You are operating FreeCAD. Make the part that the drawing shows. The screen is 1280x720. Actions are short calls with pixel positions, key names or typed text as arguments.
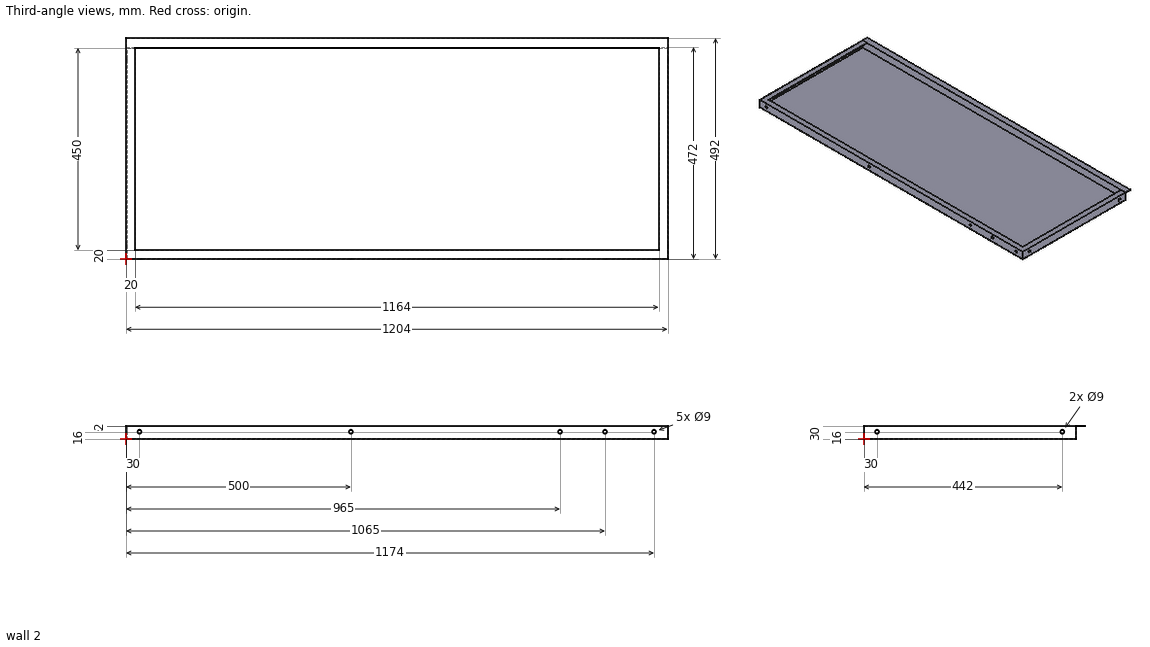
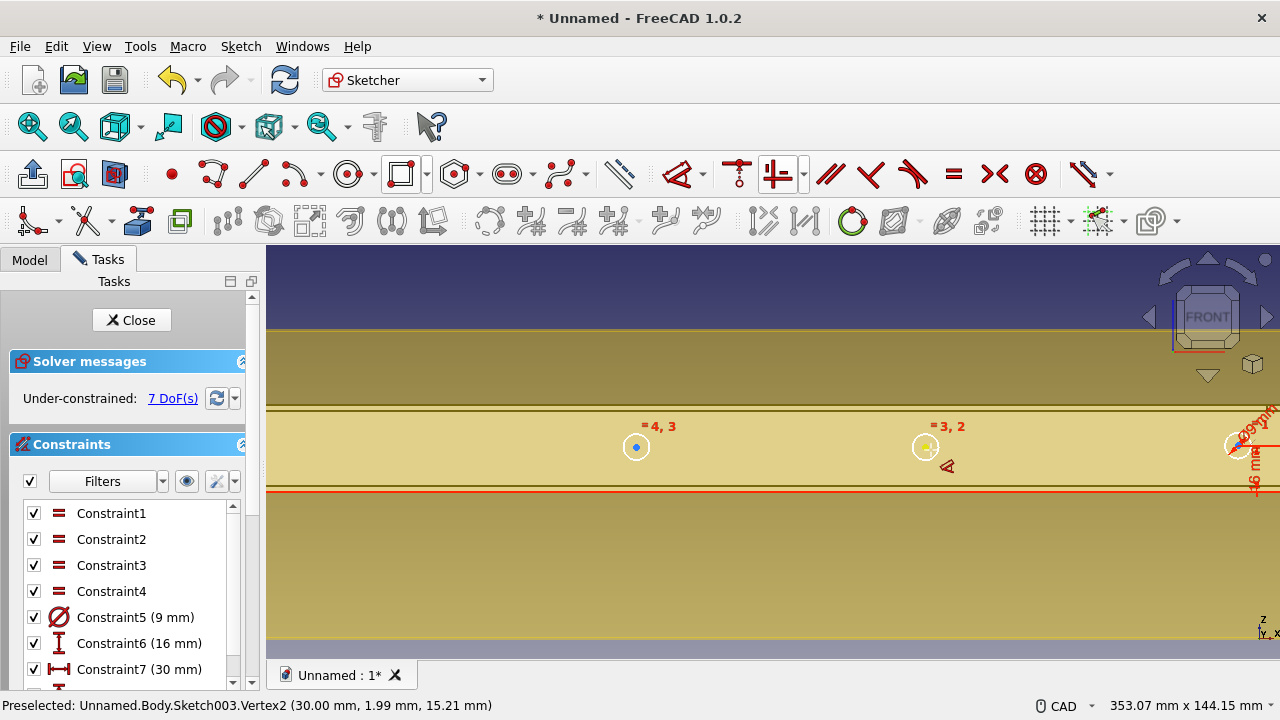
click(926, 447)
click(960, 469)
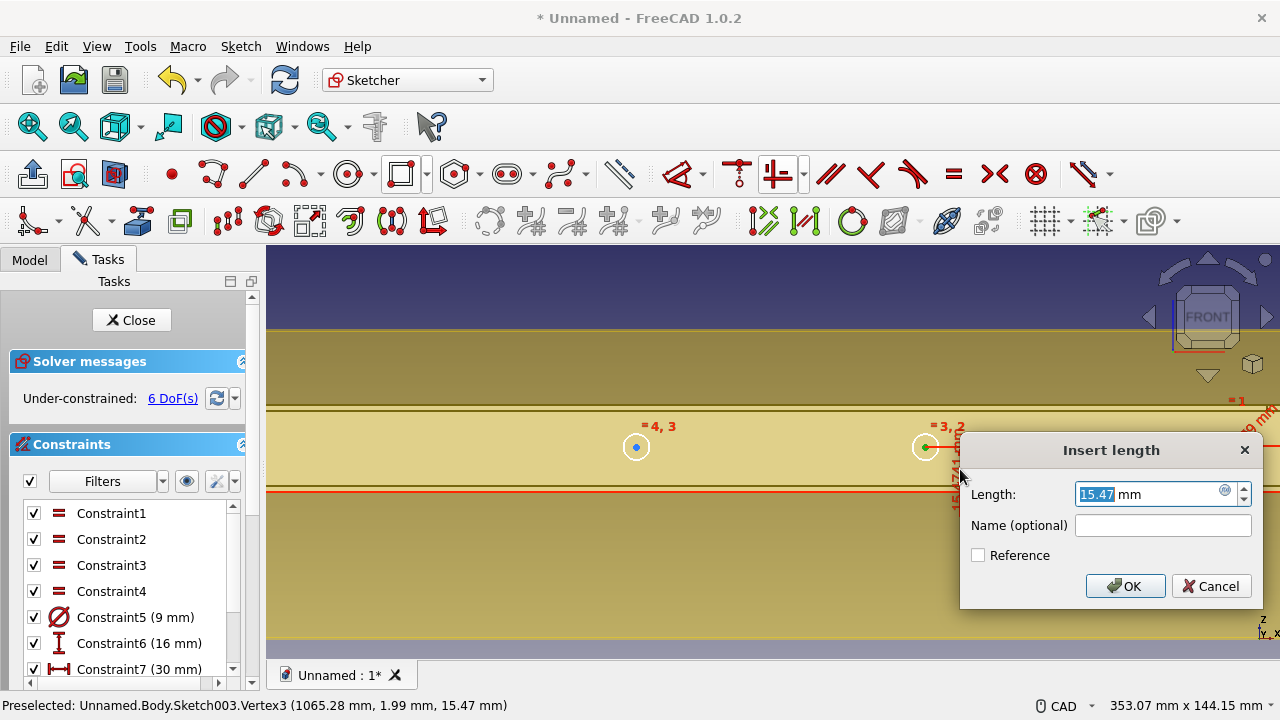
text(16)
key(Return)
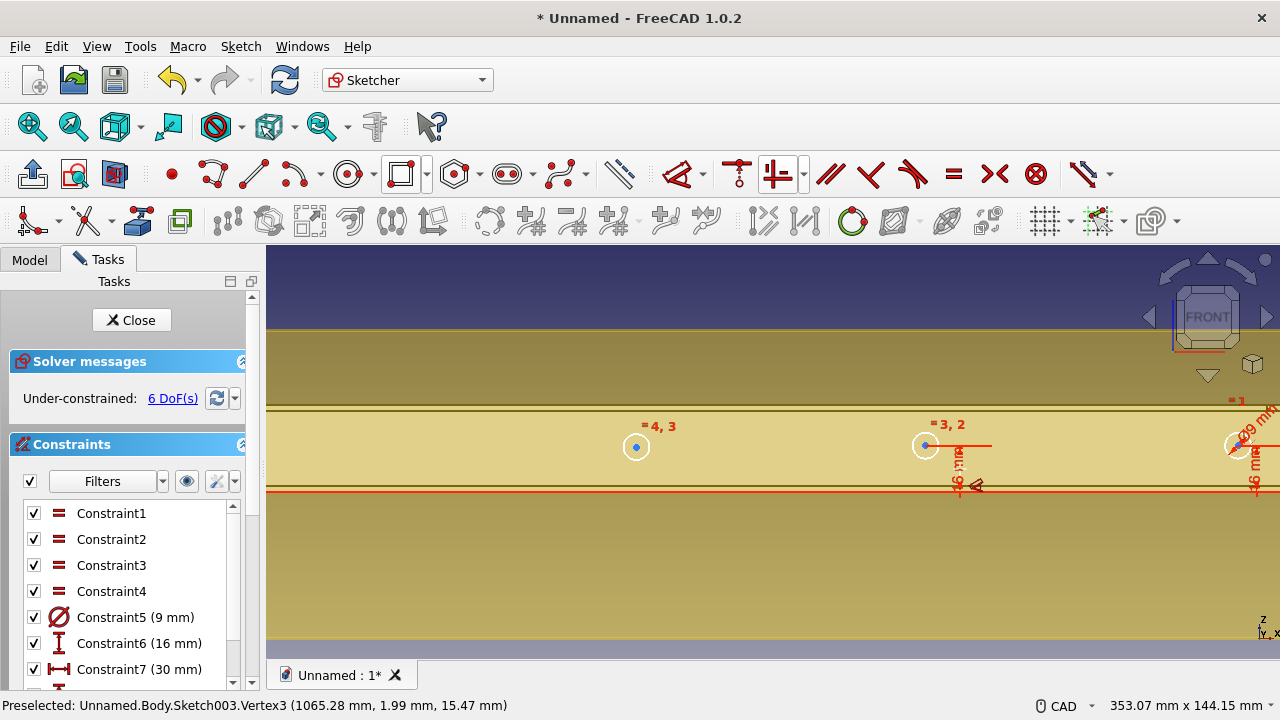
click(636, 447)
click(670, 469)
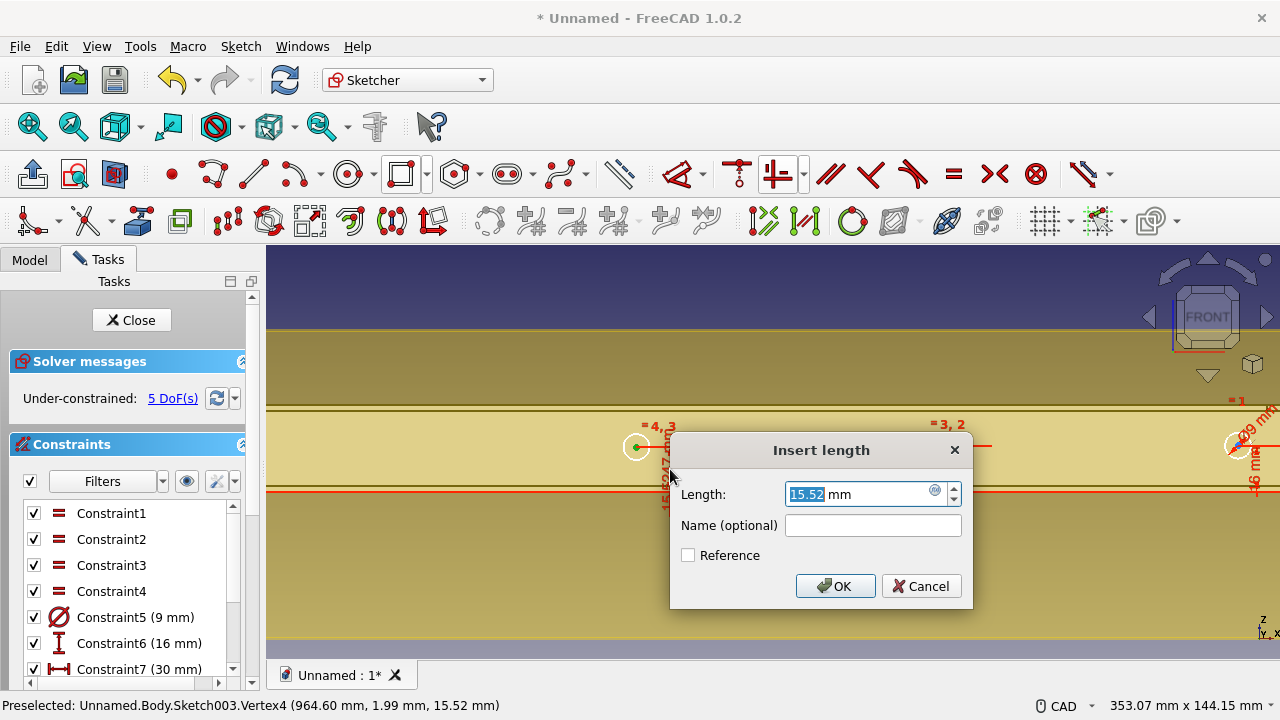
text(16)
key(Return)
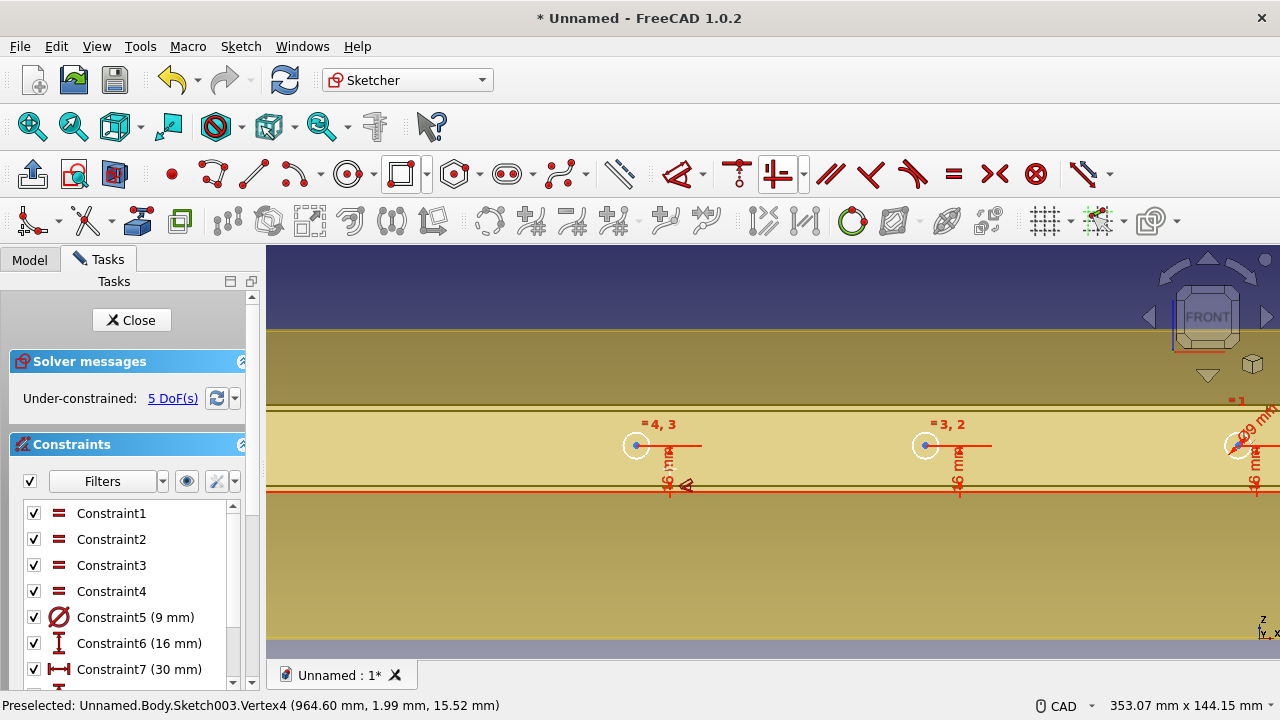
scroll(931, 450, down, 9)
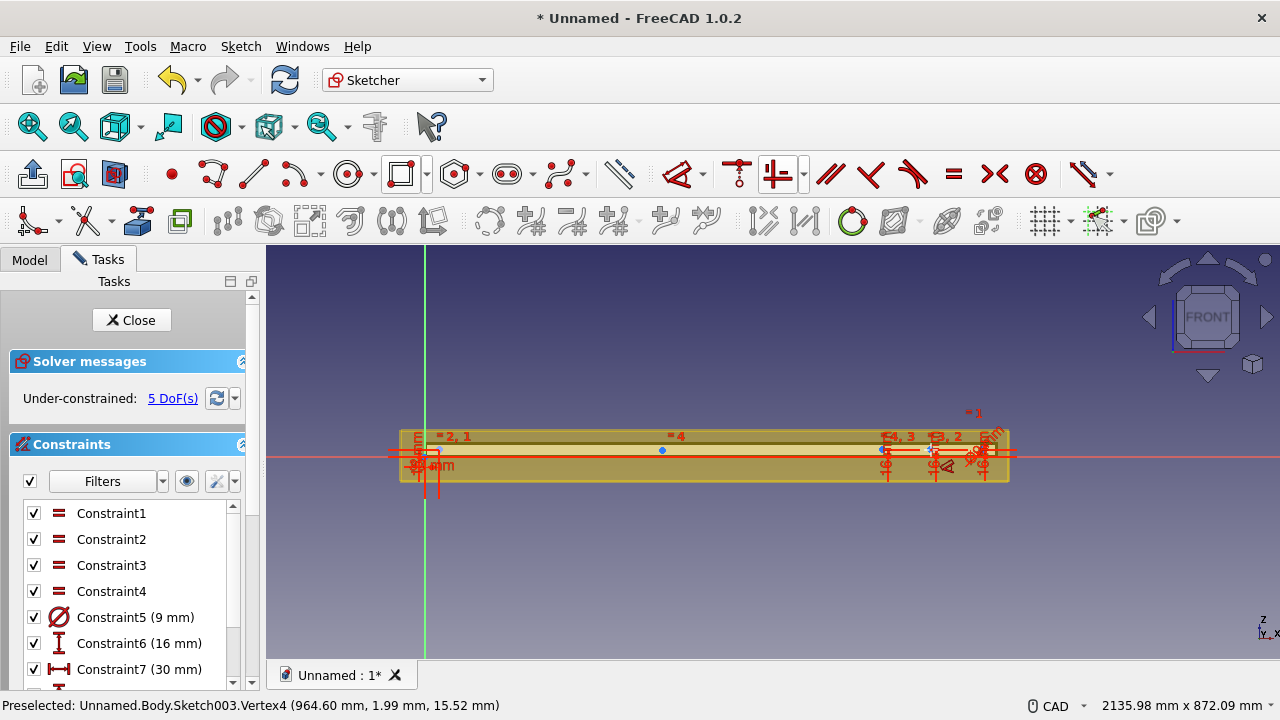
scroll(662, 450, up, 9)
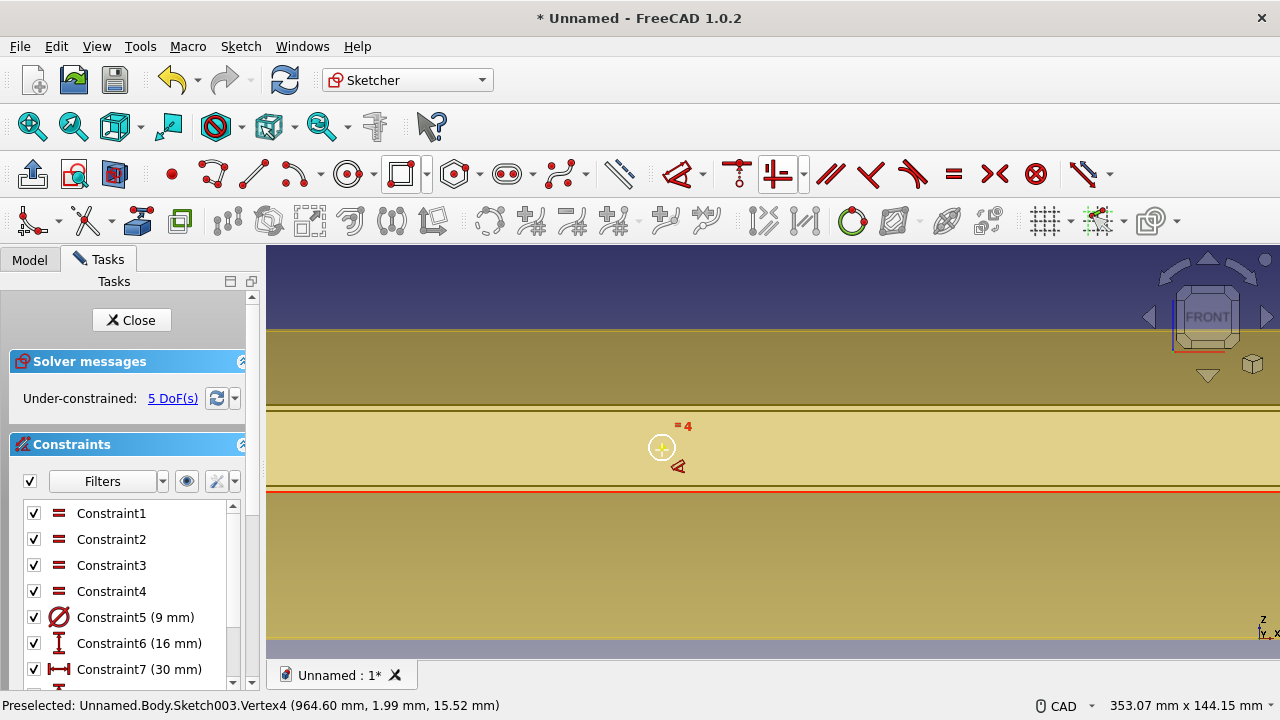
click(662, 448)
click(696, 470)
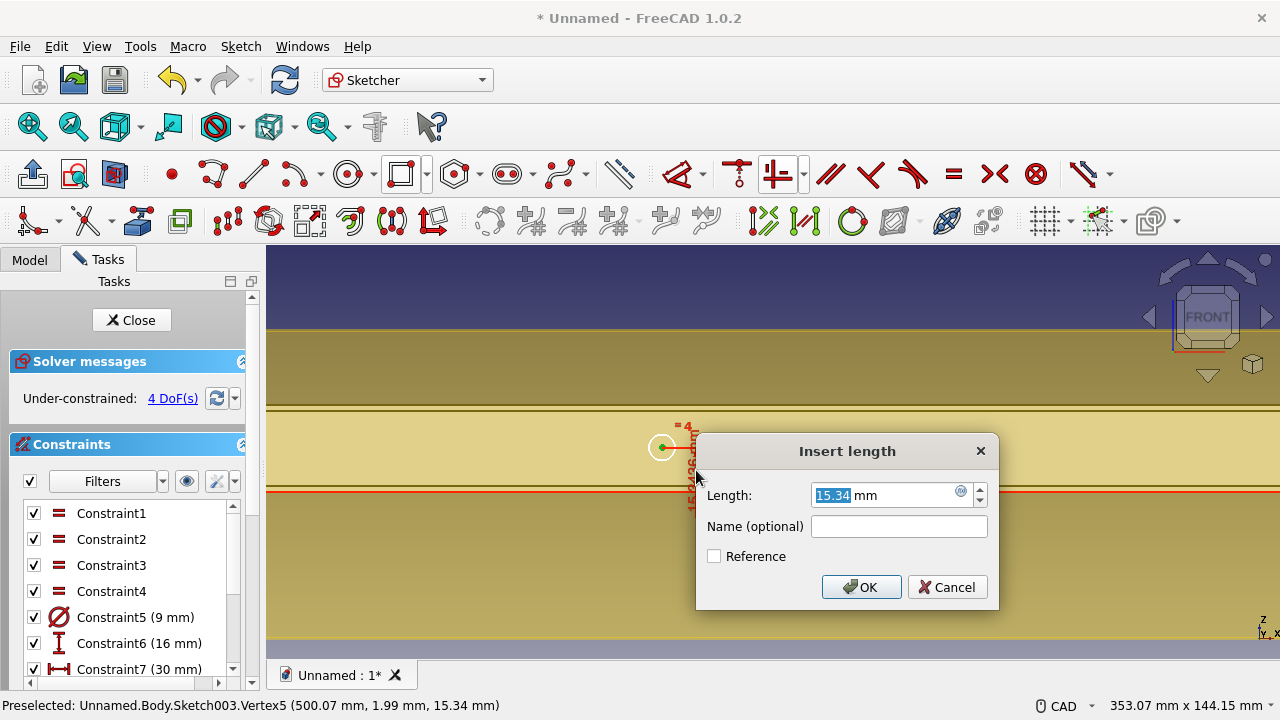
text(16)
key(Return)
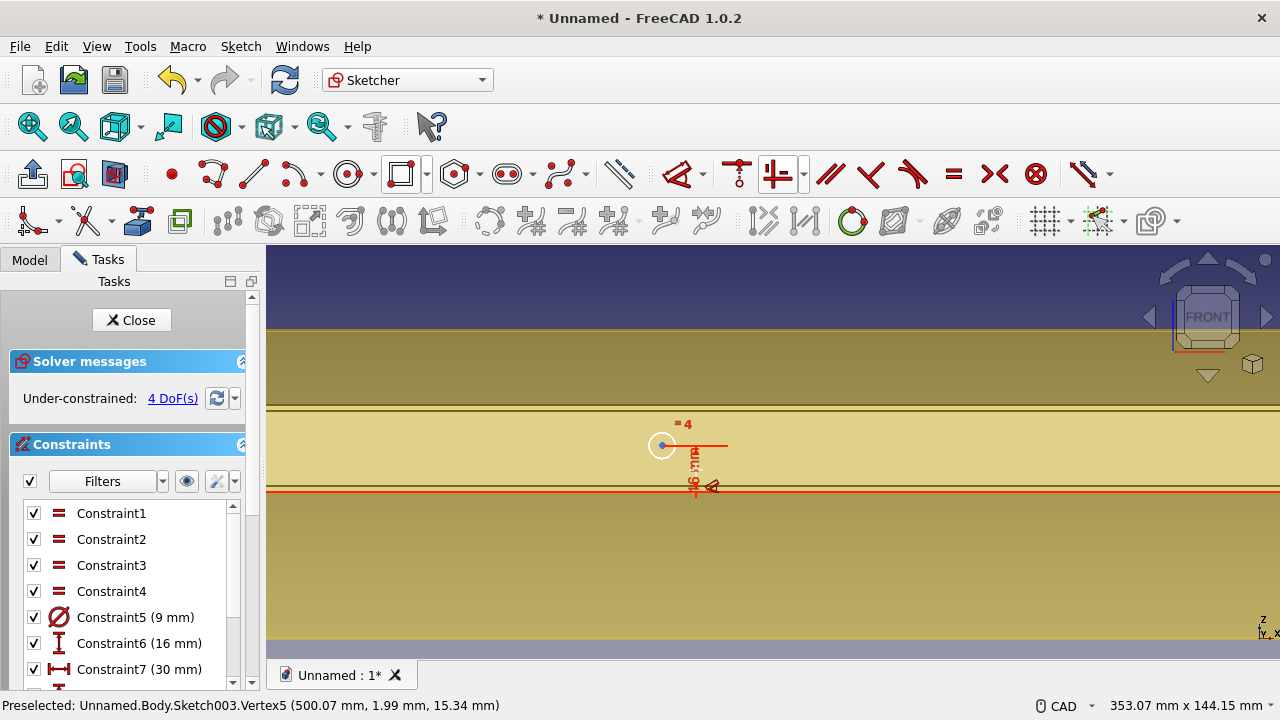
scroll(662, 450, down, 9)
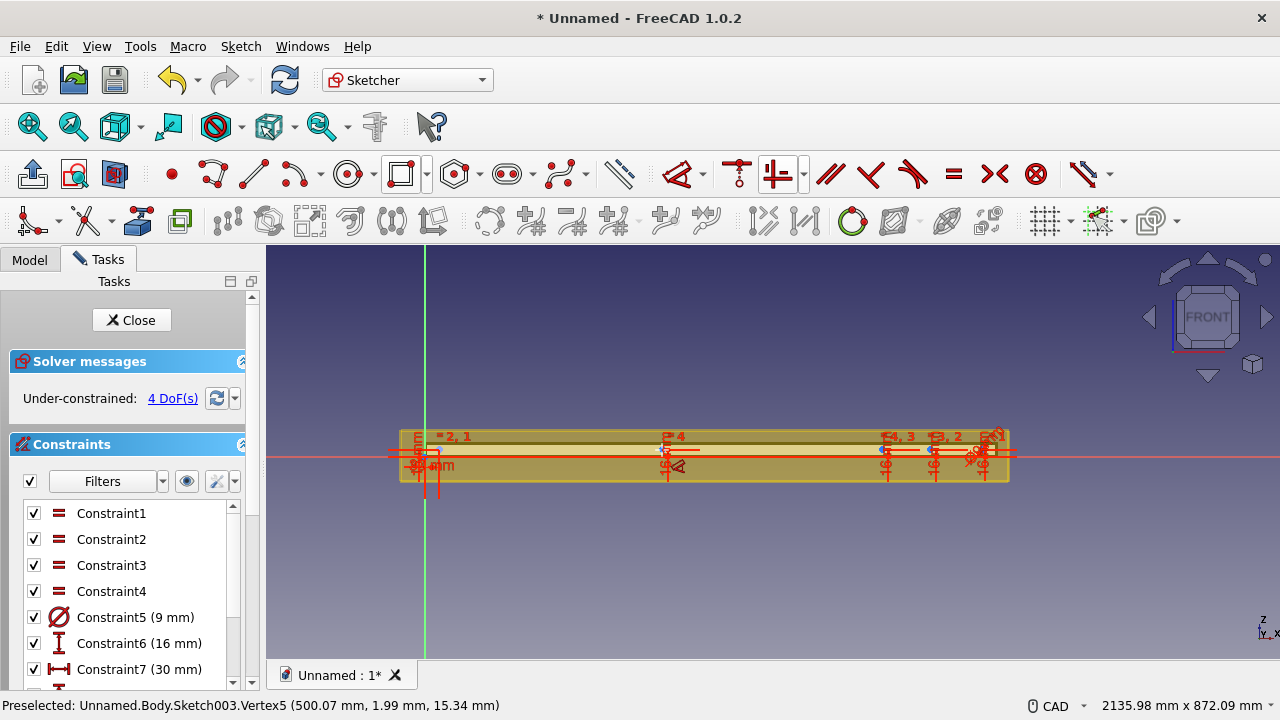
click(883, 450)
click(654, 491)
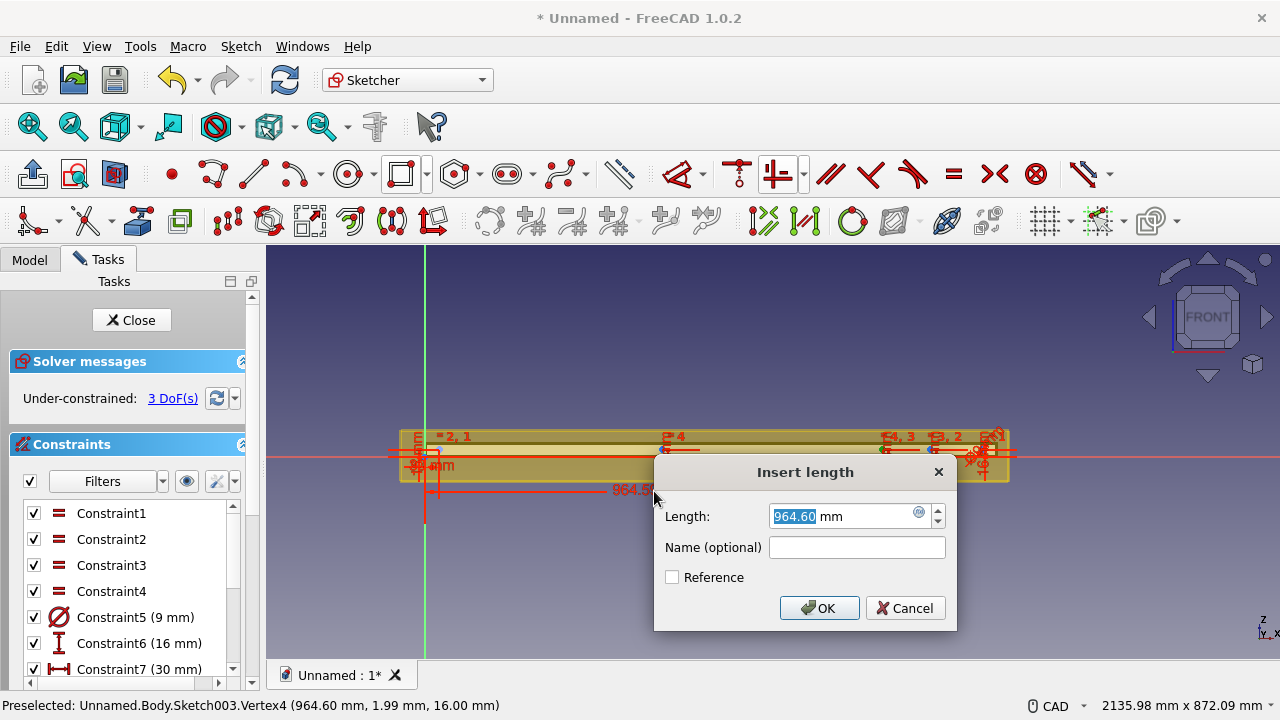
text(965)
key(Return)